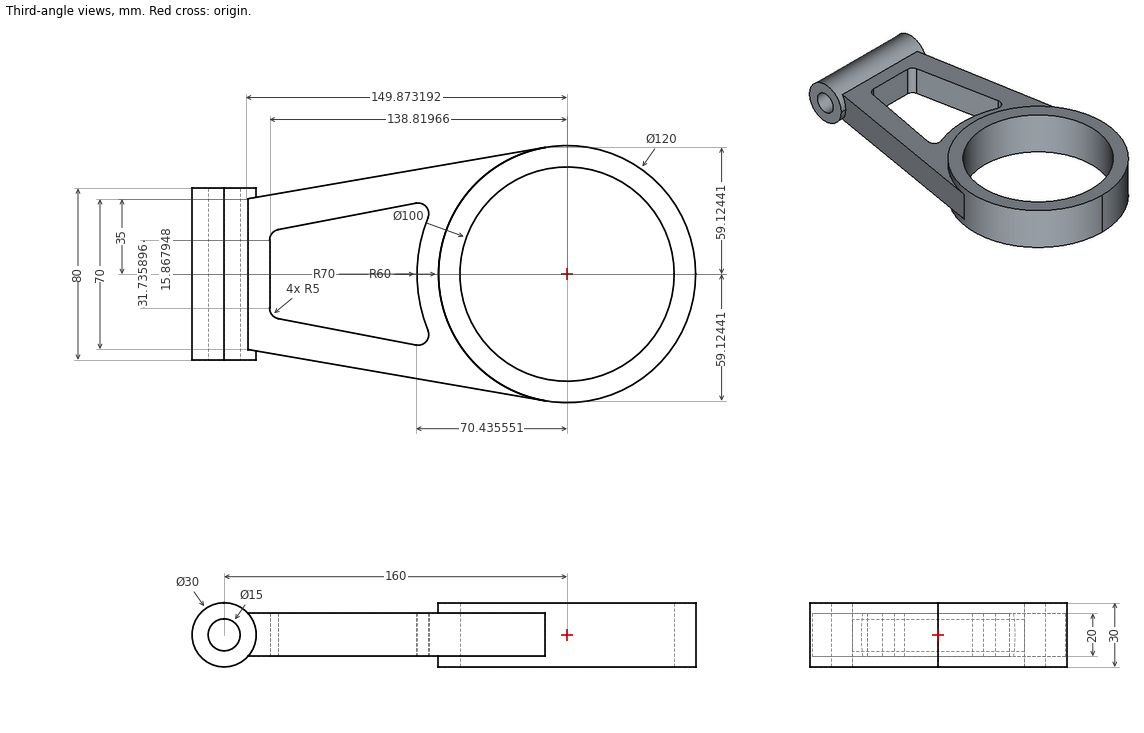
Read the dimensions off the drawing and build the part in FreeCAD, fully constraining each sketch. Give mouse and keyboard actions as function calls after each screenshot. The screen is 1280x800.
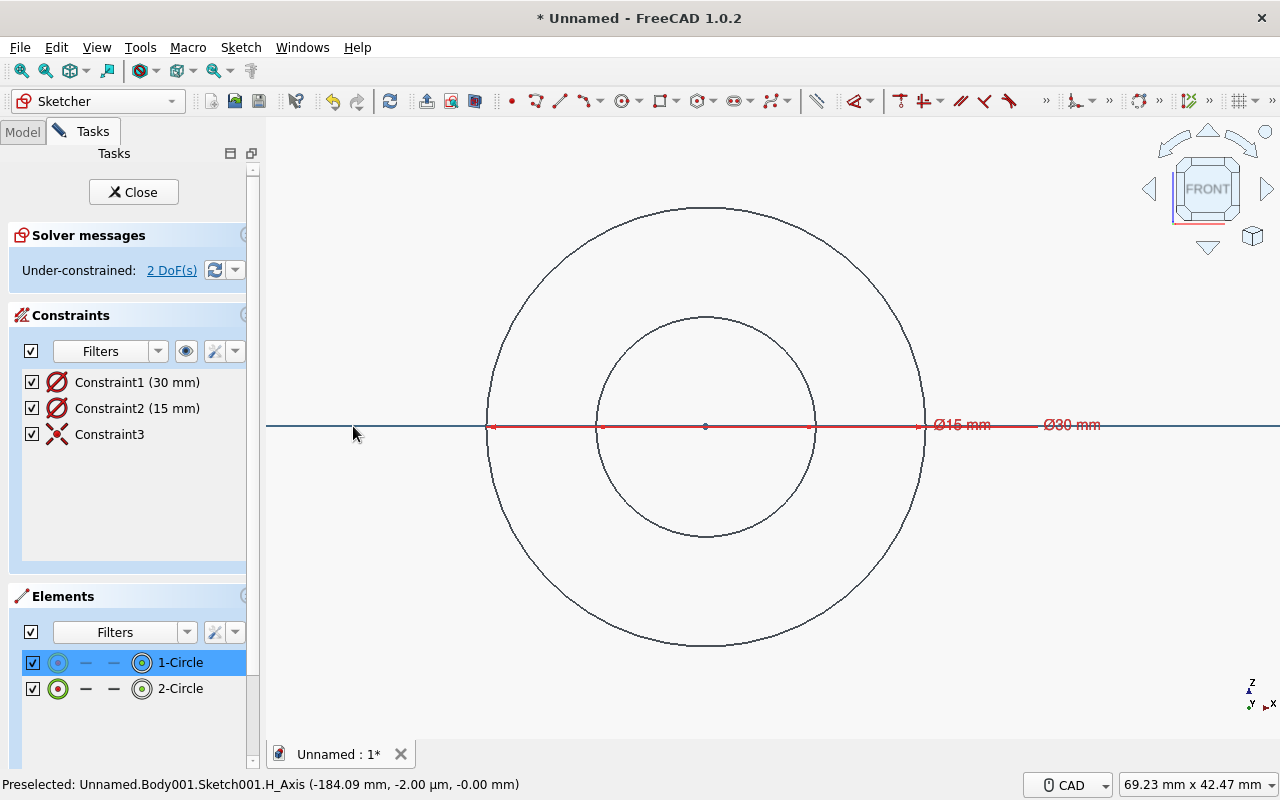
click(900, 102)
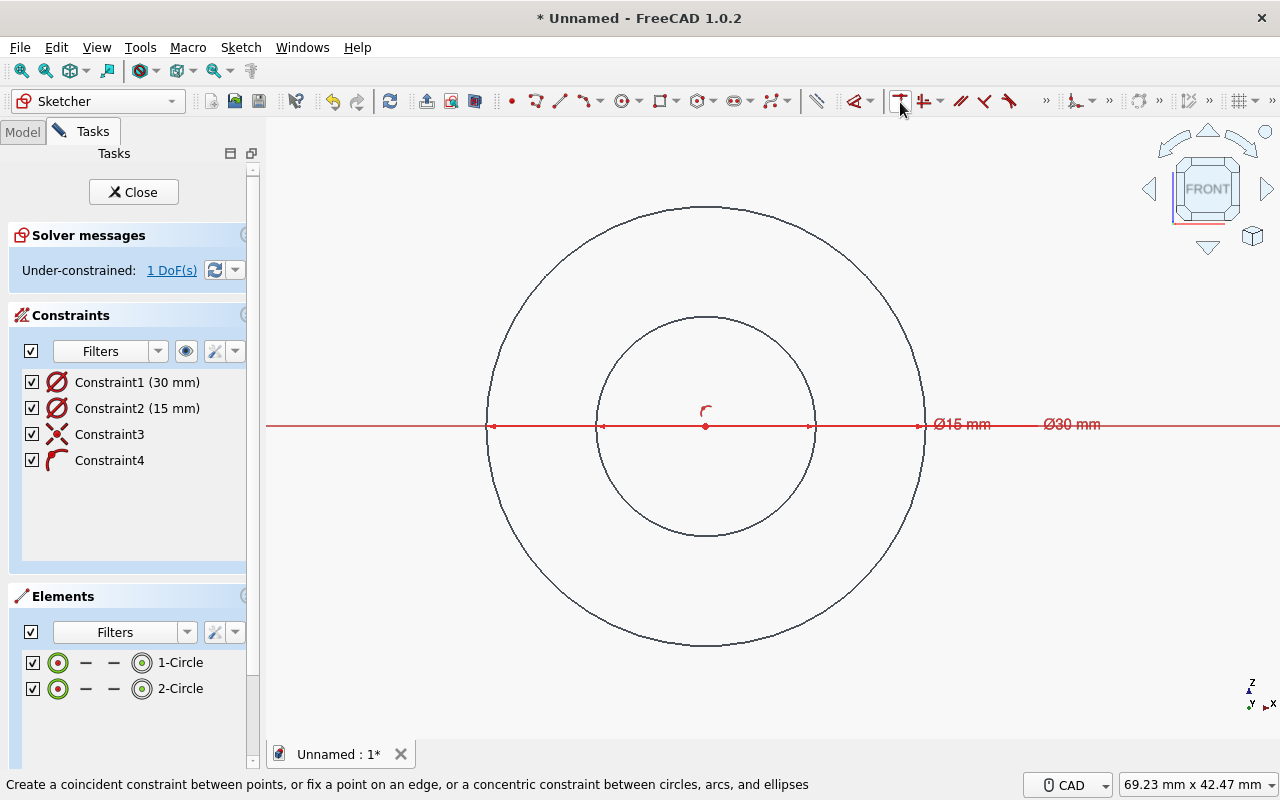
click(854, 102)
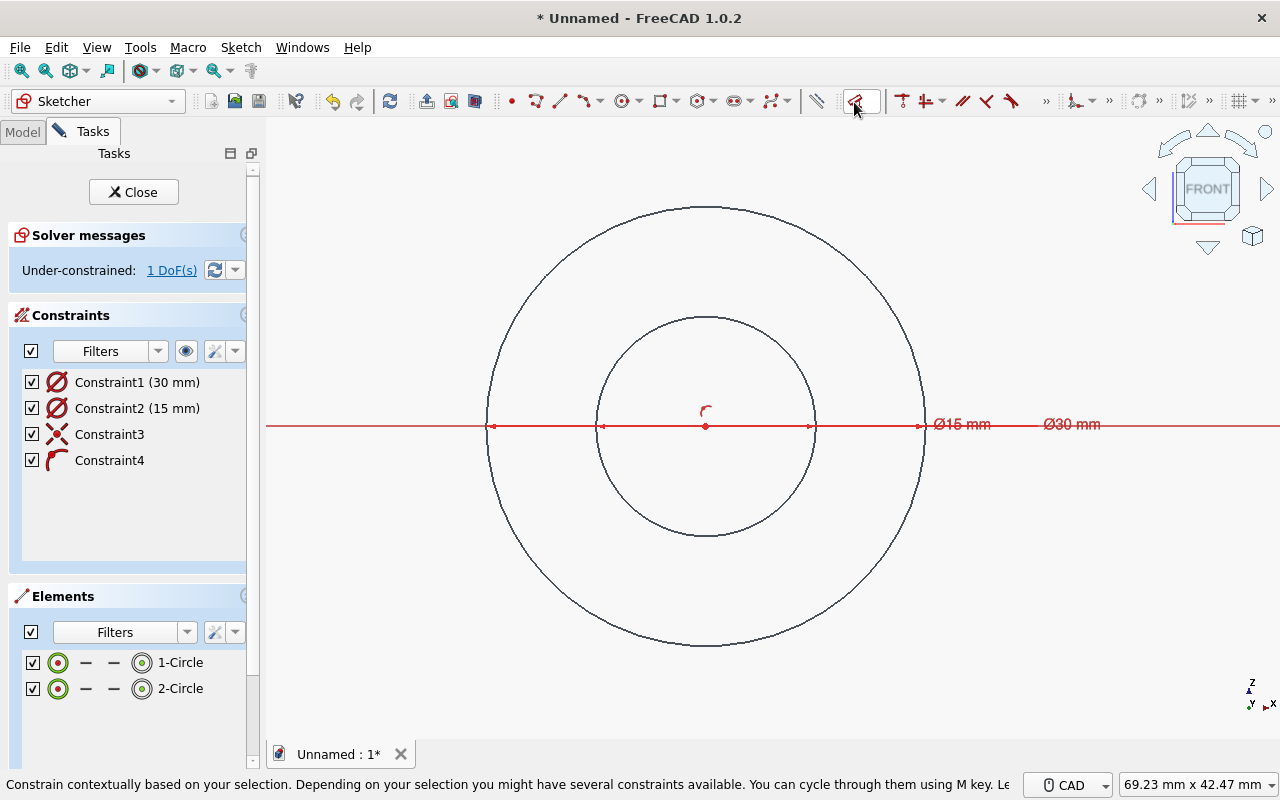
click(706, 426)
click(1005, 460)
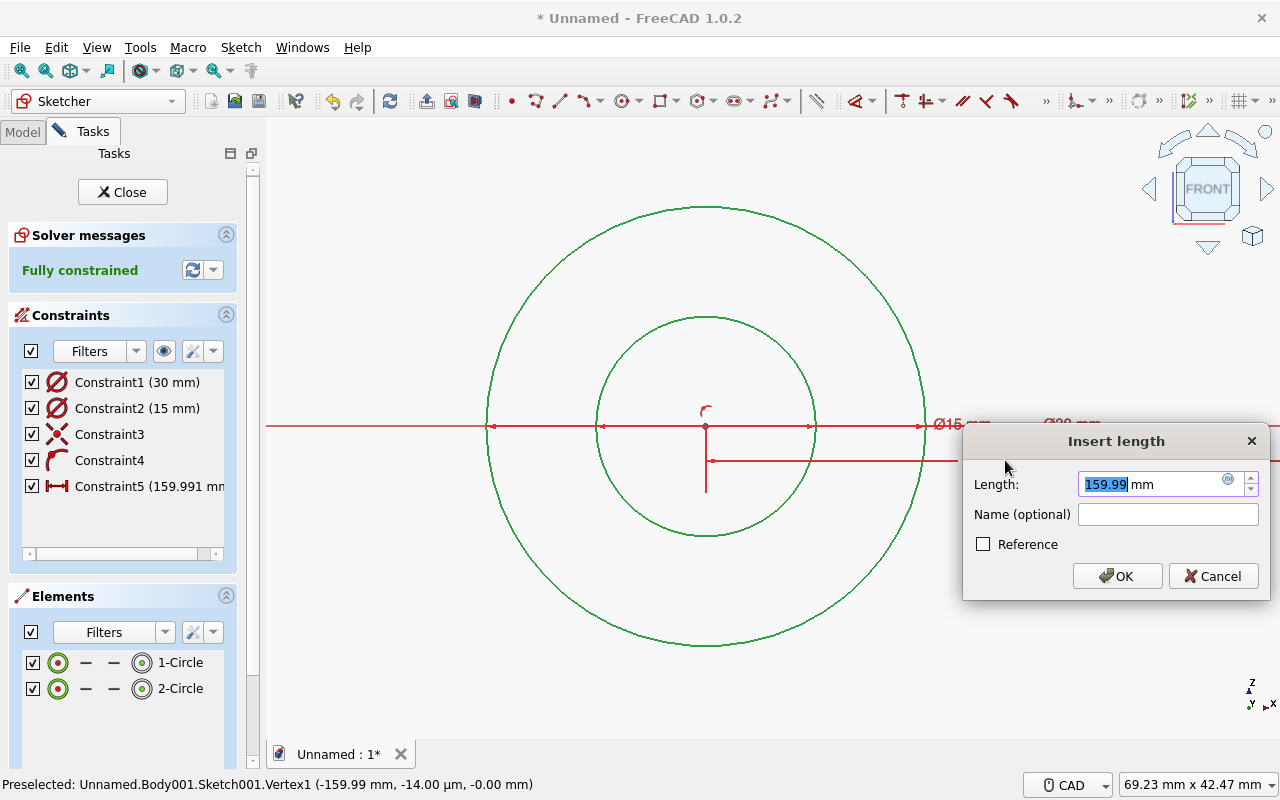
text(160)
key(Return)
key(Escape)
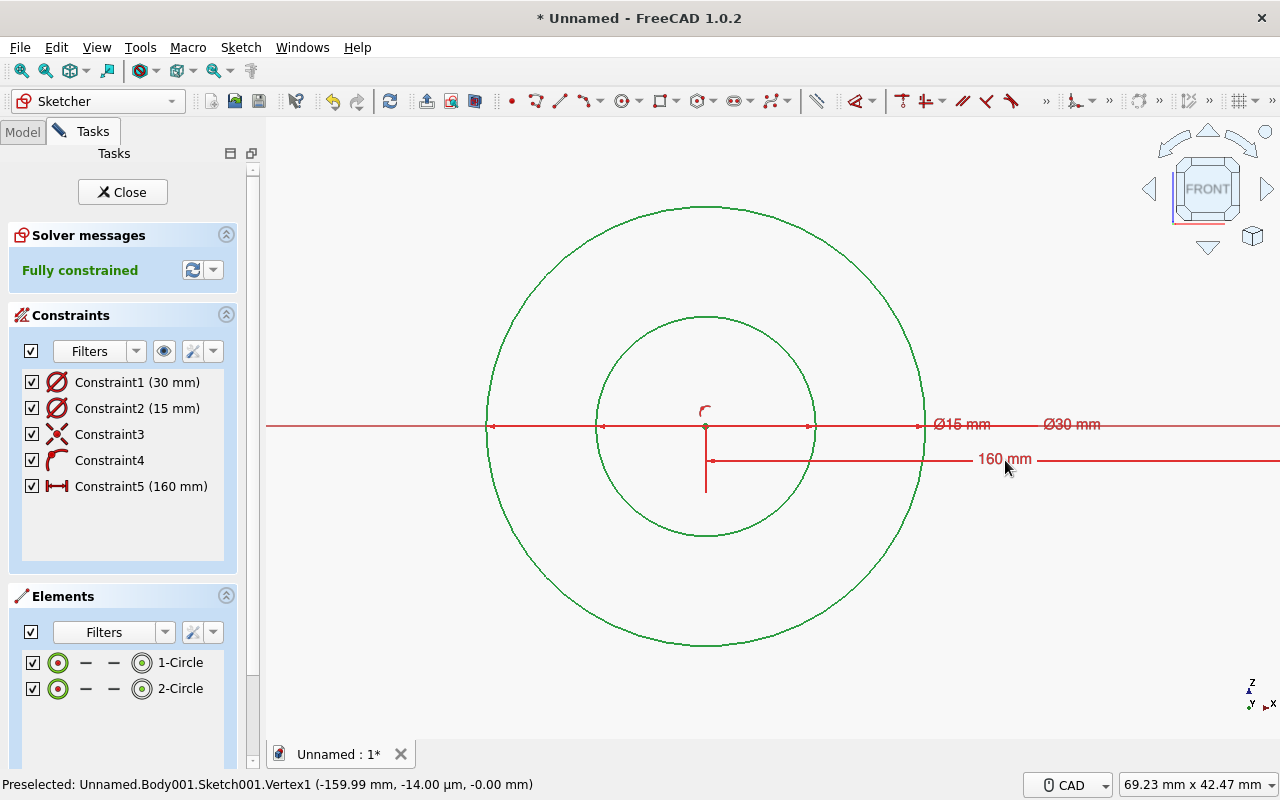
click(123, 192)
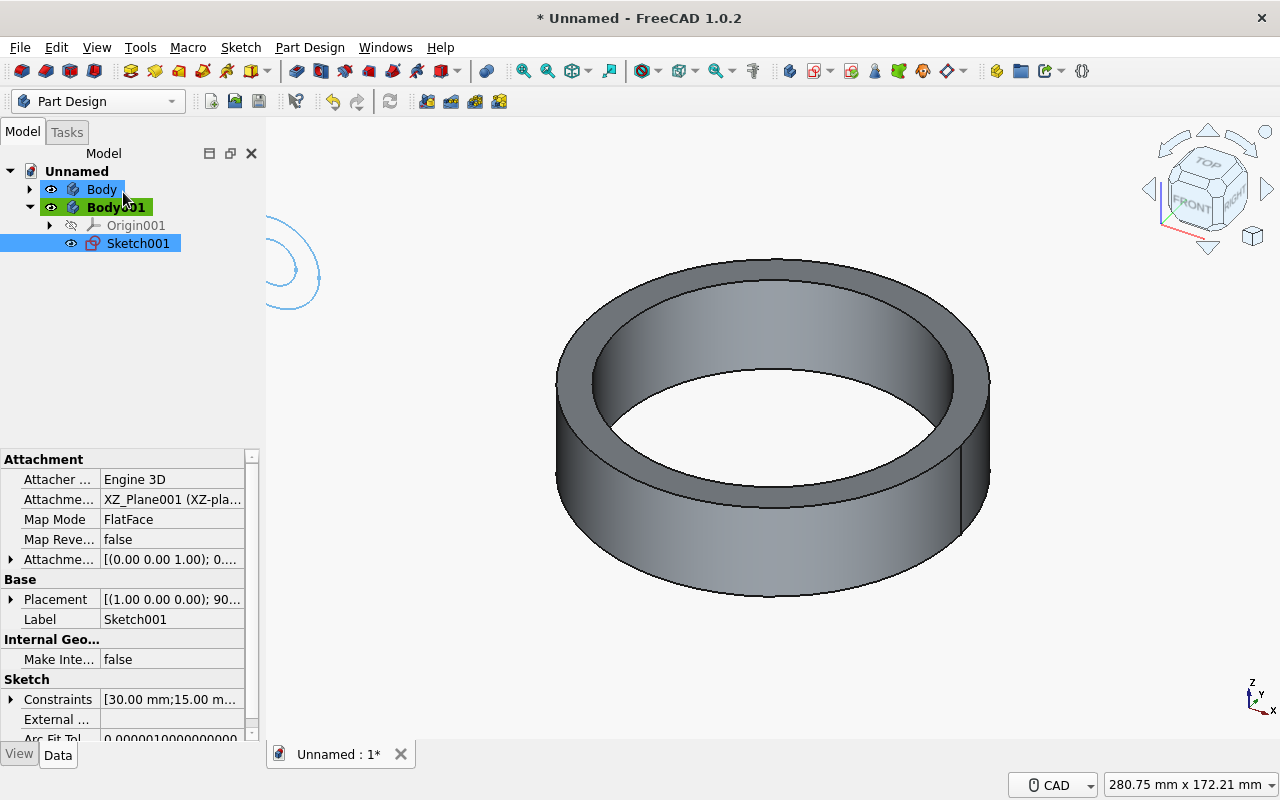
click(132, 72)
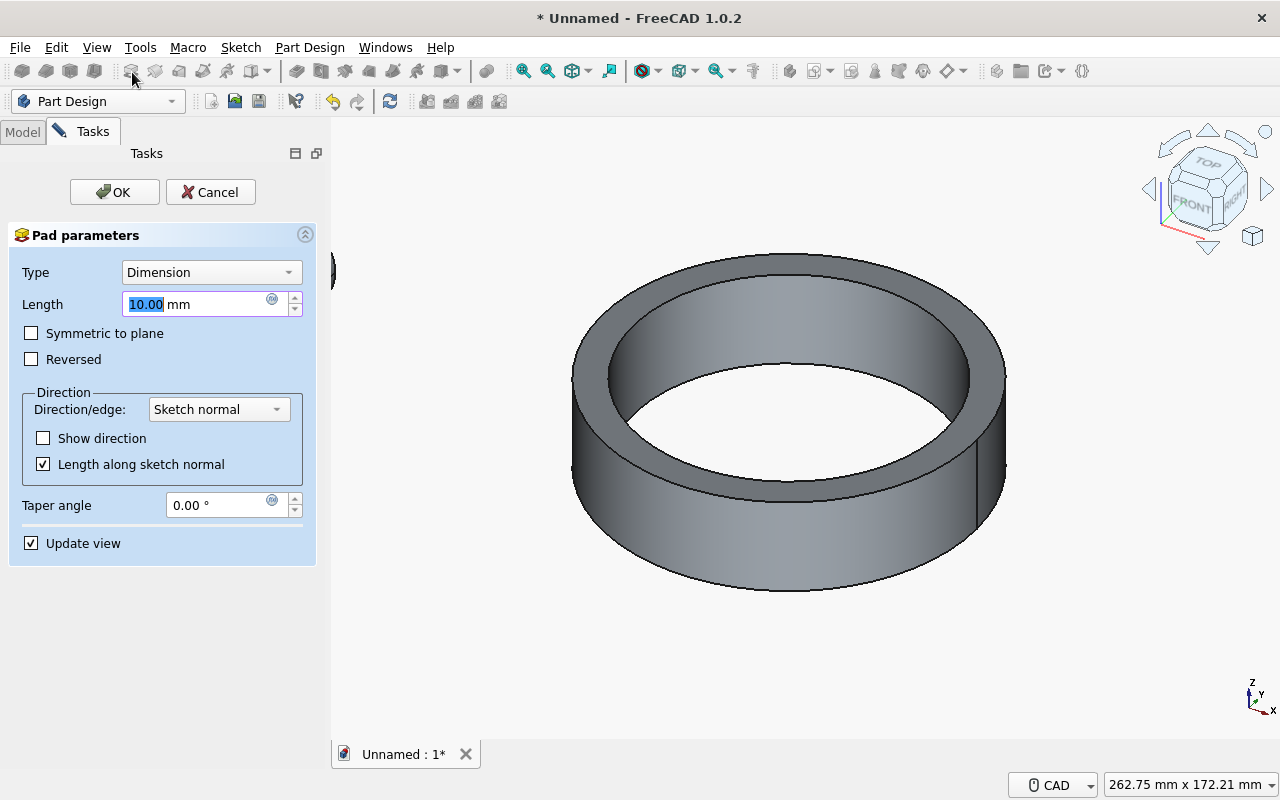
text(80)
key(Tab)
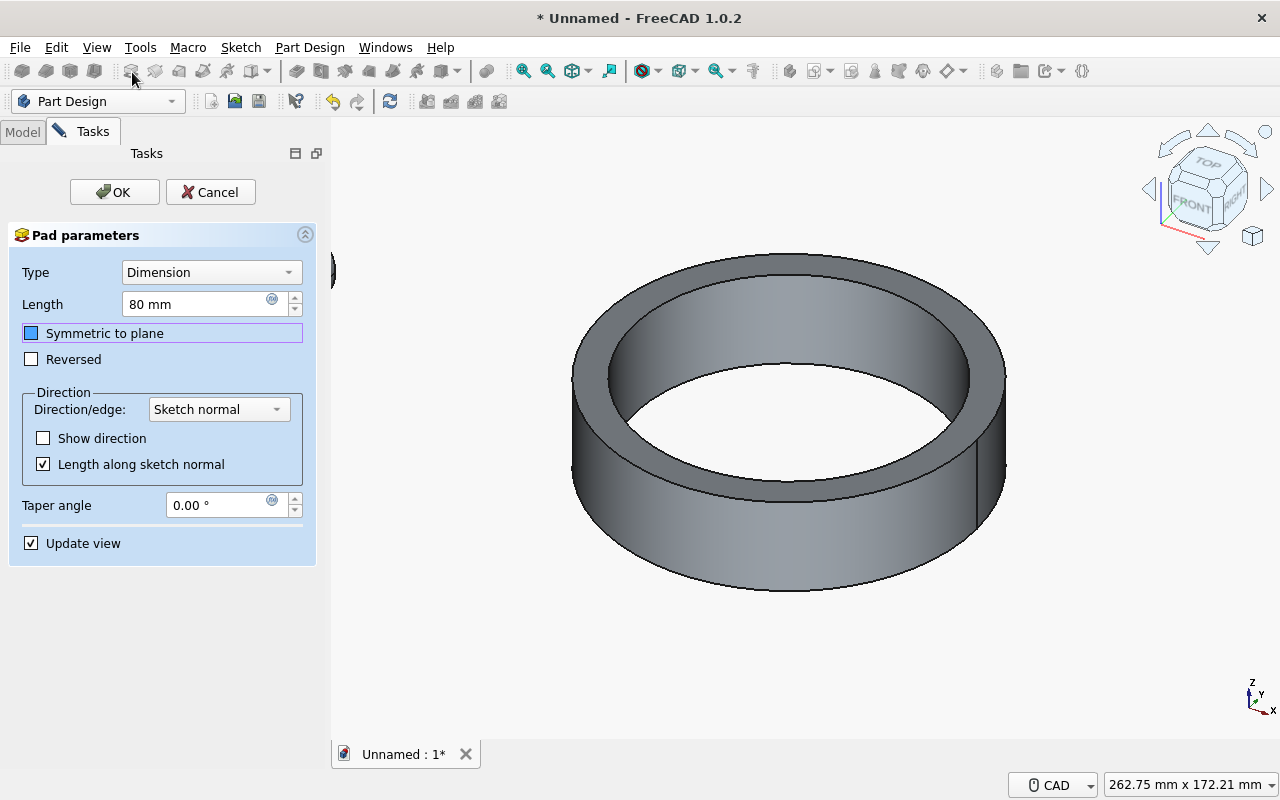
click(30, 333)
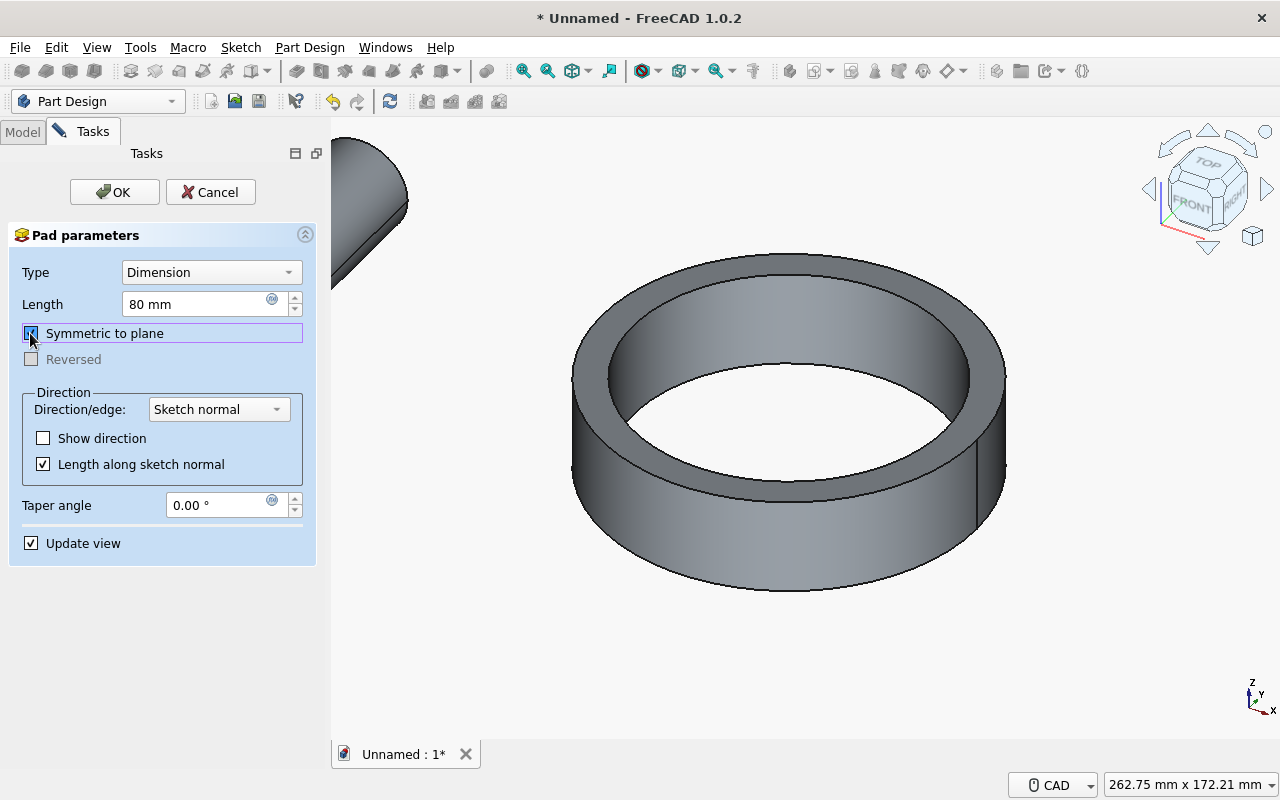
click(115, 192)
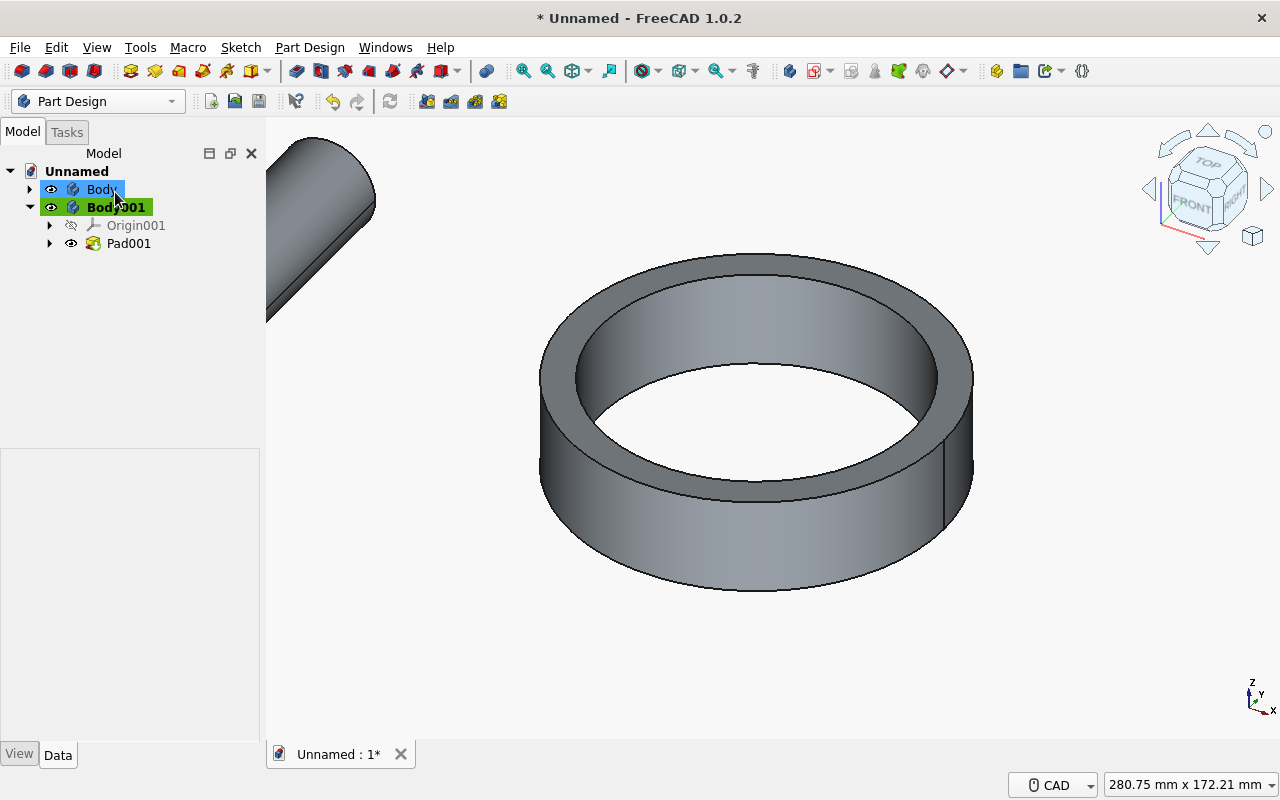
click(524, 72)